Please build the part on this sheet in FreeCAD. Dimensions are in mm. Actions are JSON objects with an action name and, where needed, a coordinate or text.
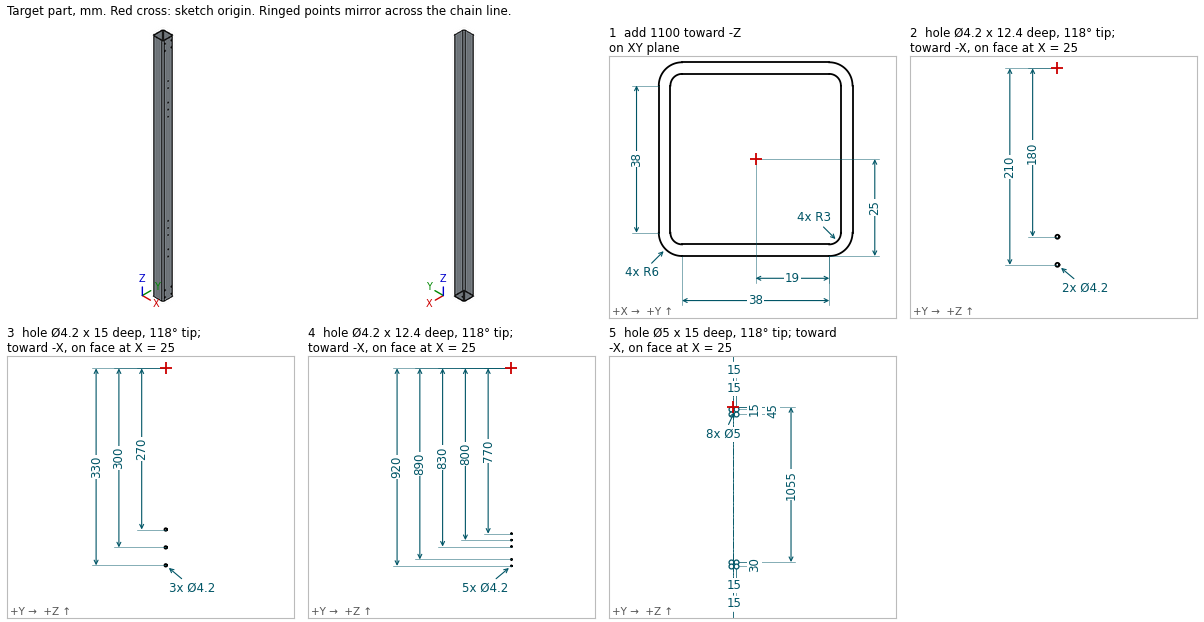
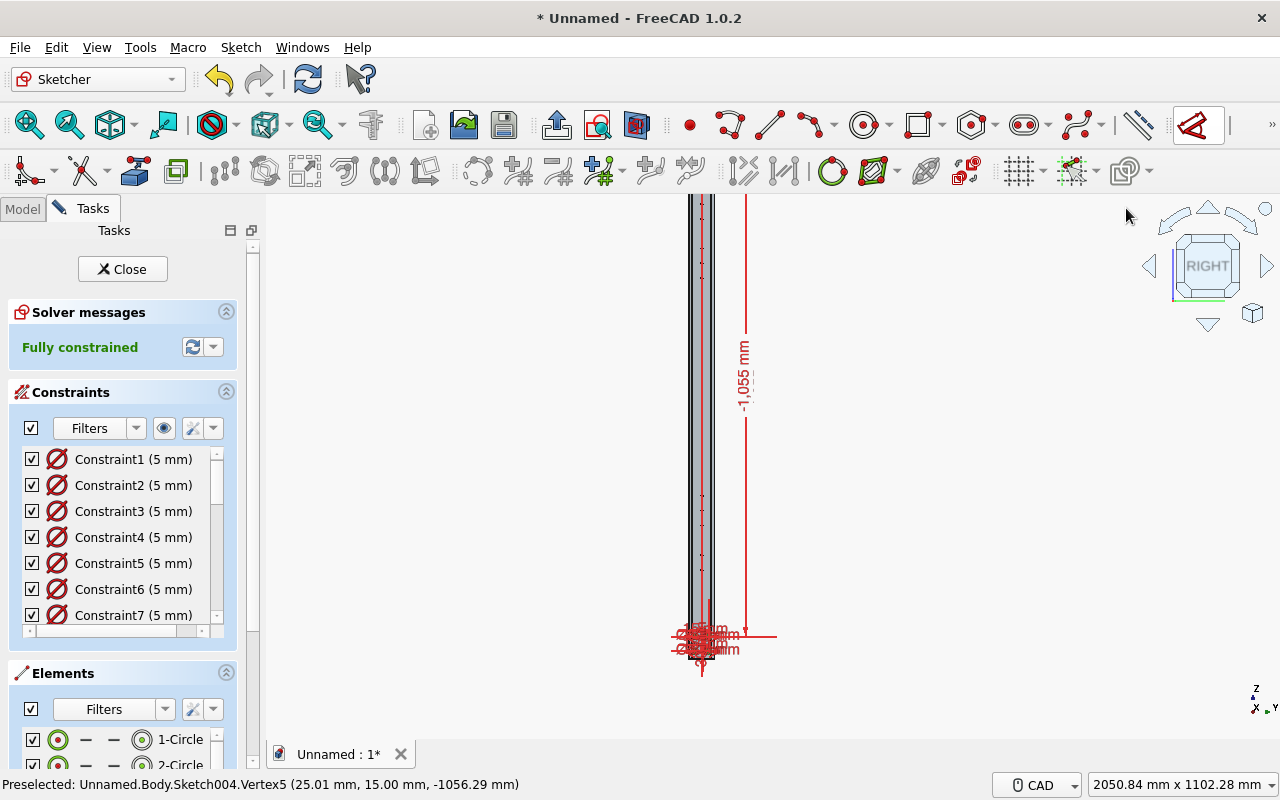
{"action": "left_click", "coordinate": [123, 269]}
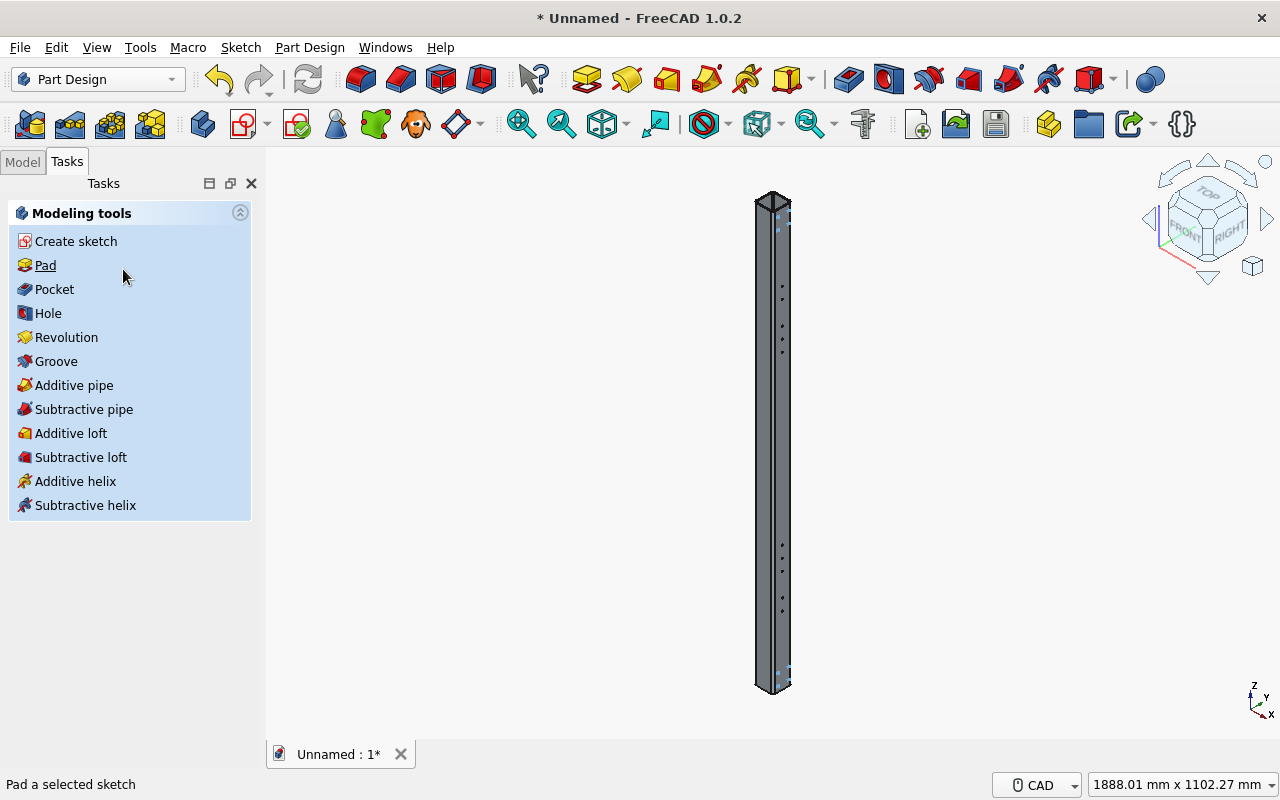
{"action": "left_click", "coordinate": [890, 80]}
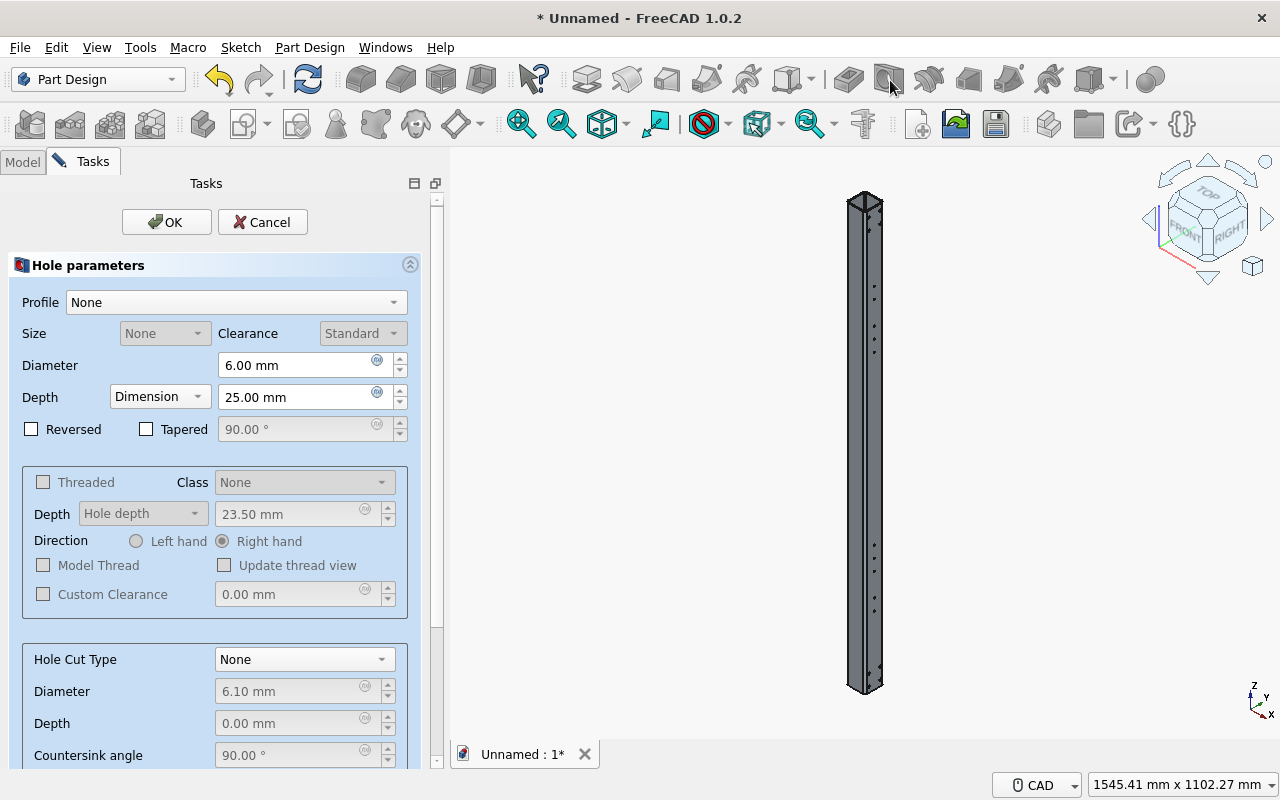
{"action": "triple_click", "coordinate": [305, 365]}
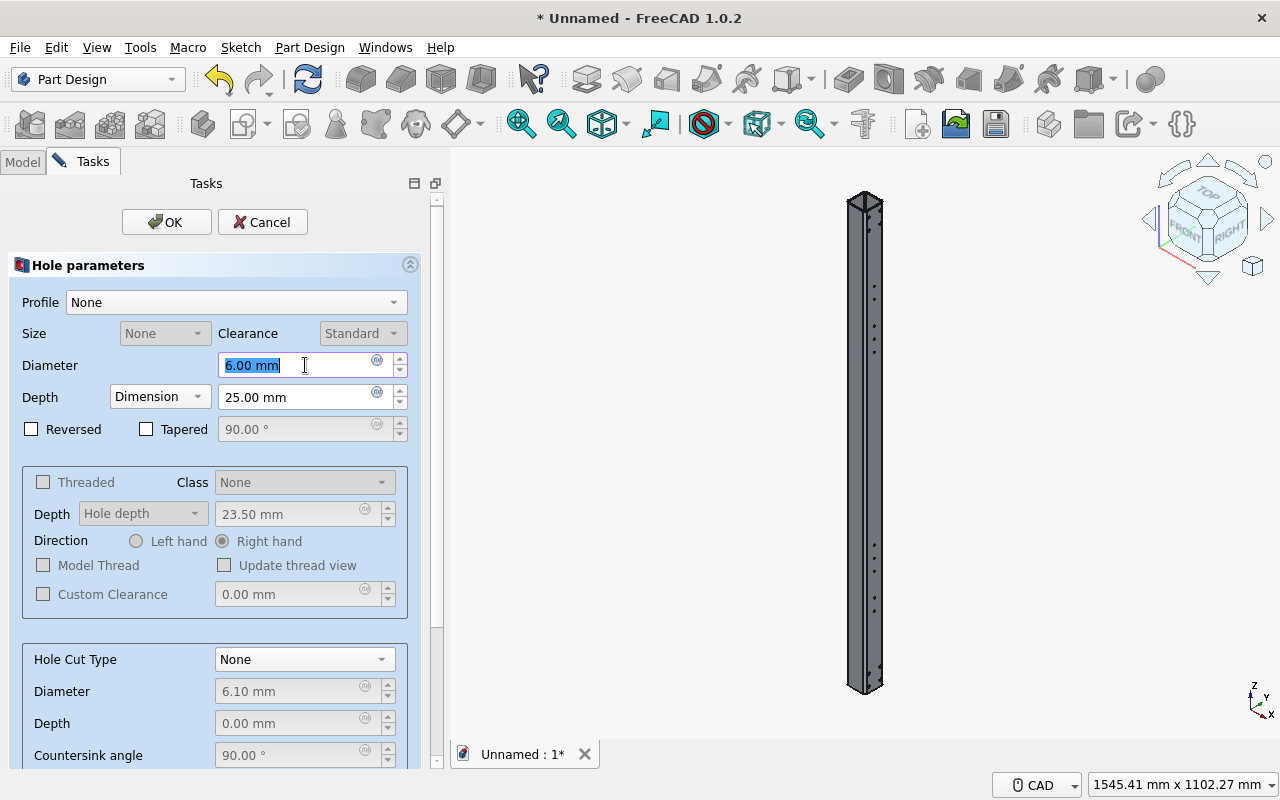
{"action": "type", "text": "5"}
{"action": "key", "text": "Tab"}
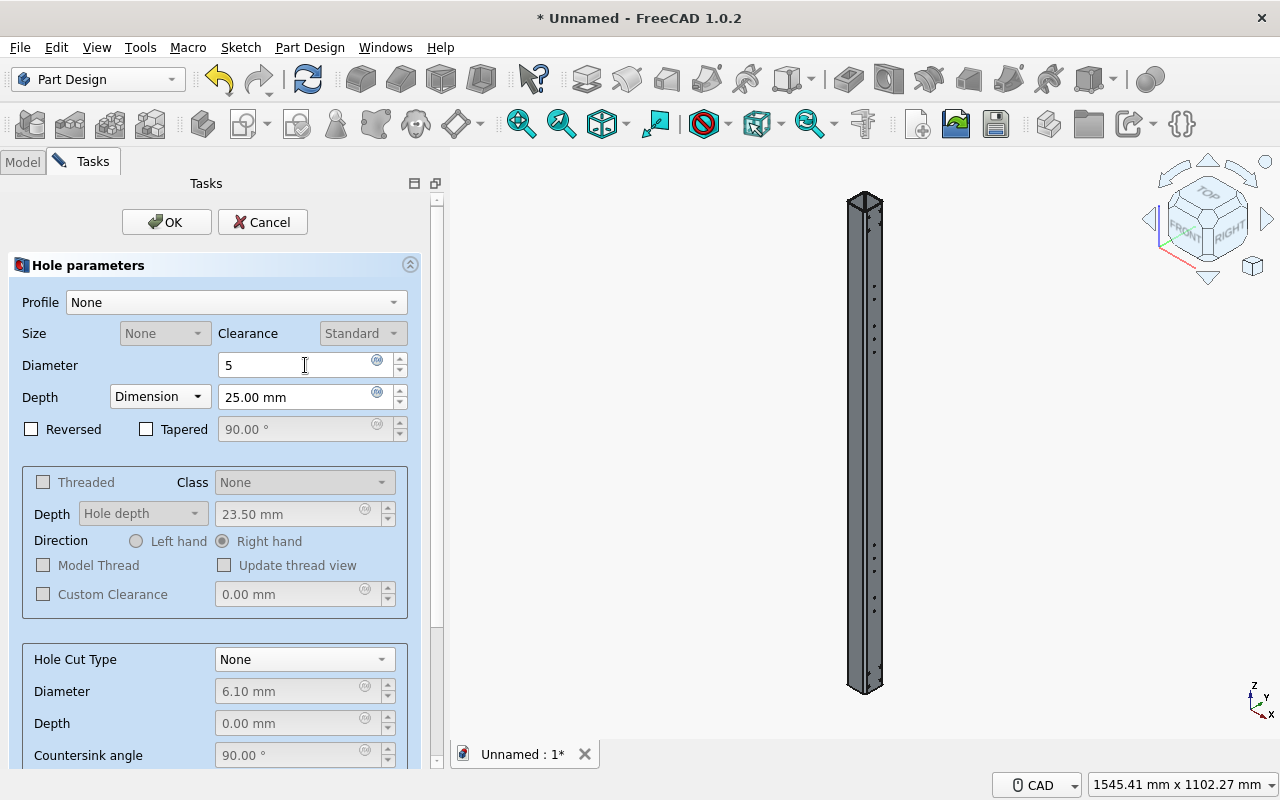
{"action": "triple_click", "coordinate": [305, 397]}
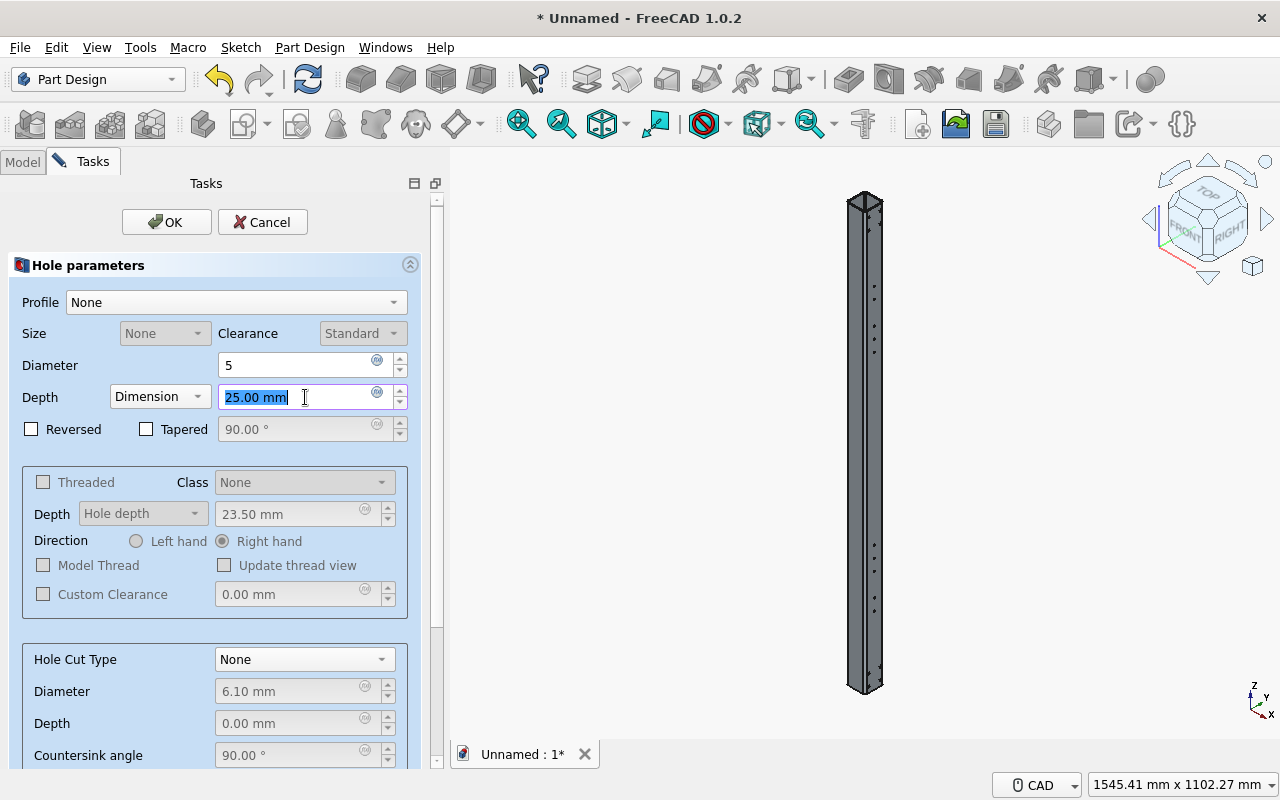
{"action": "type", "text": "15"}
{"action": "key", "text": "Tab"}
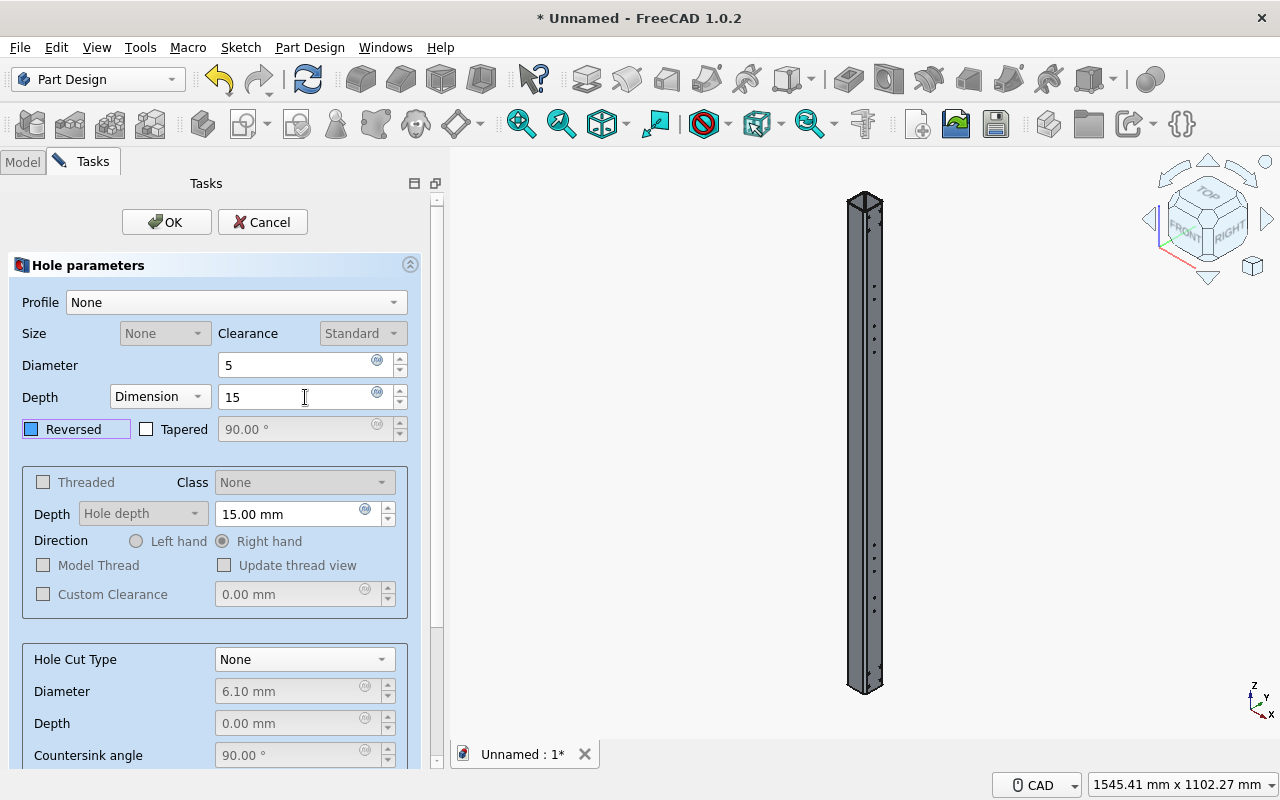
{"action": "left_click", "coordinate": [167, 222]}